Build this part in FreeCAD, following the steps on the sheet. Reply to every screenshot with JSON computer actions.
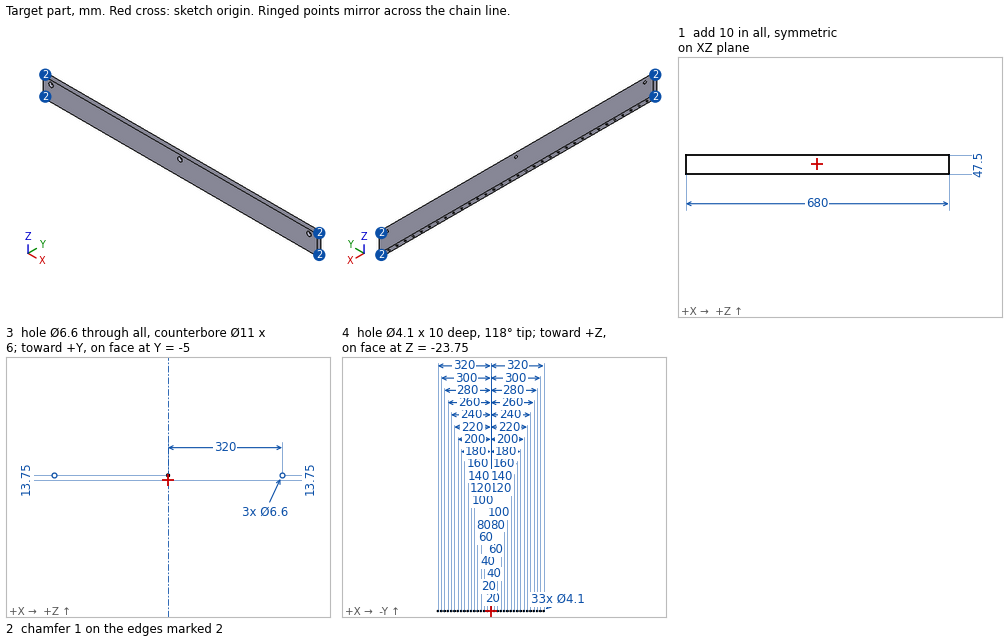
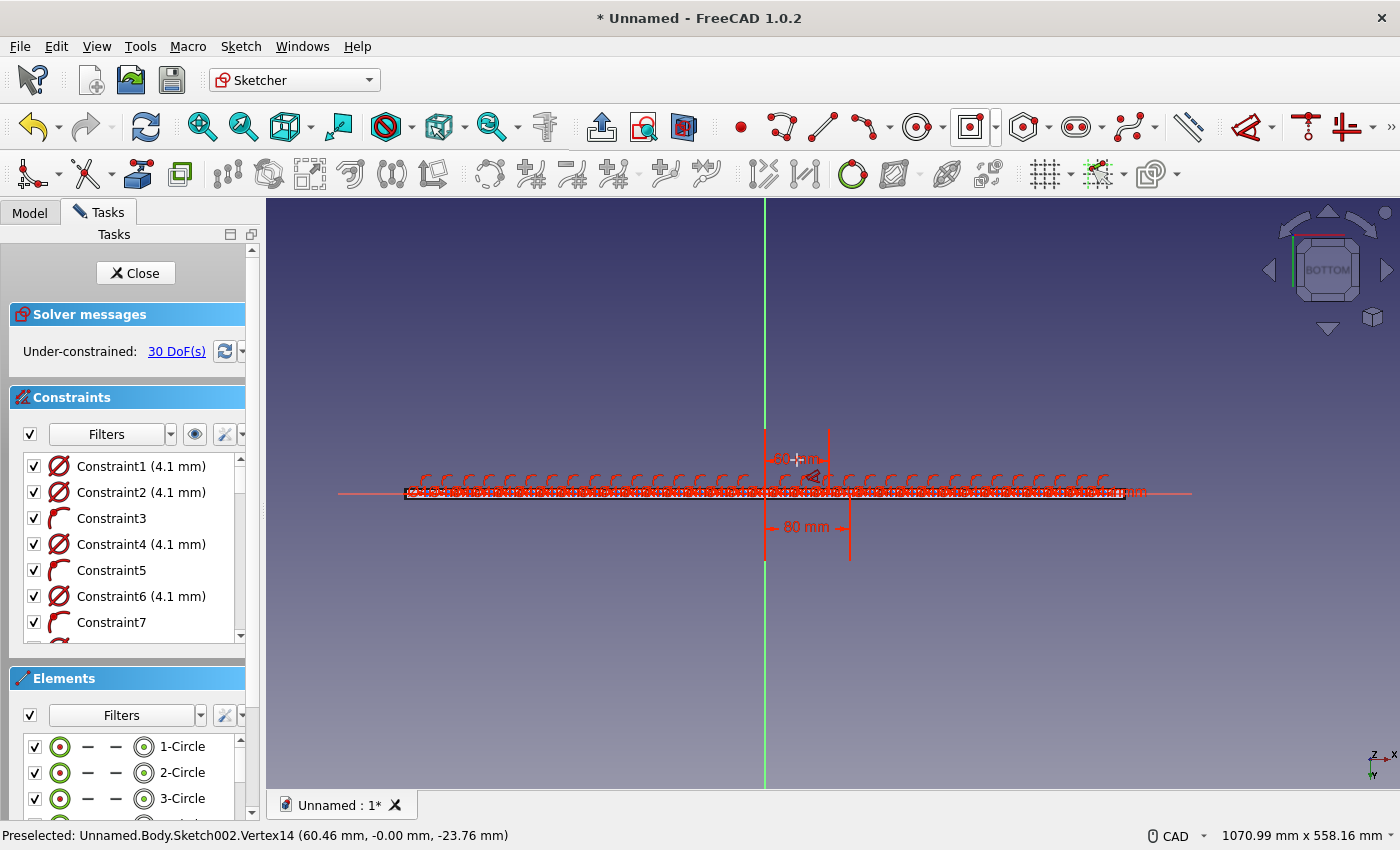
{"action": "left_click", "coordinate": [807, 494]}
{"action": "left_click", "coordinate": [786, 552]}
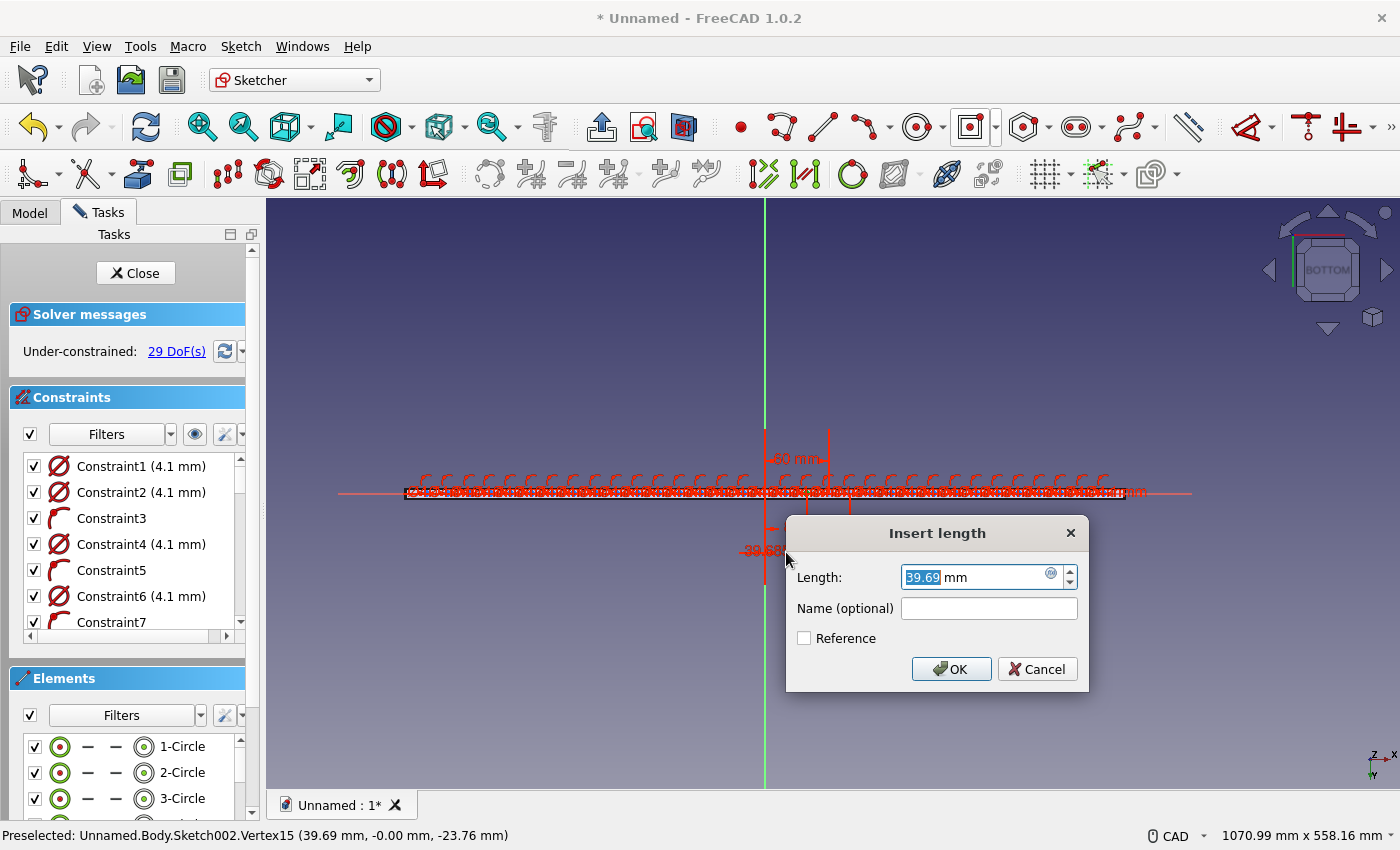
{"action": "type", "text": "40"}
{"action": "key", "text": "Return"}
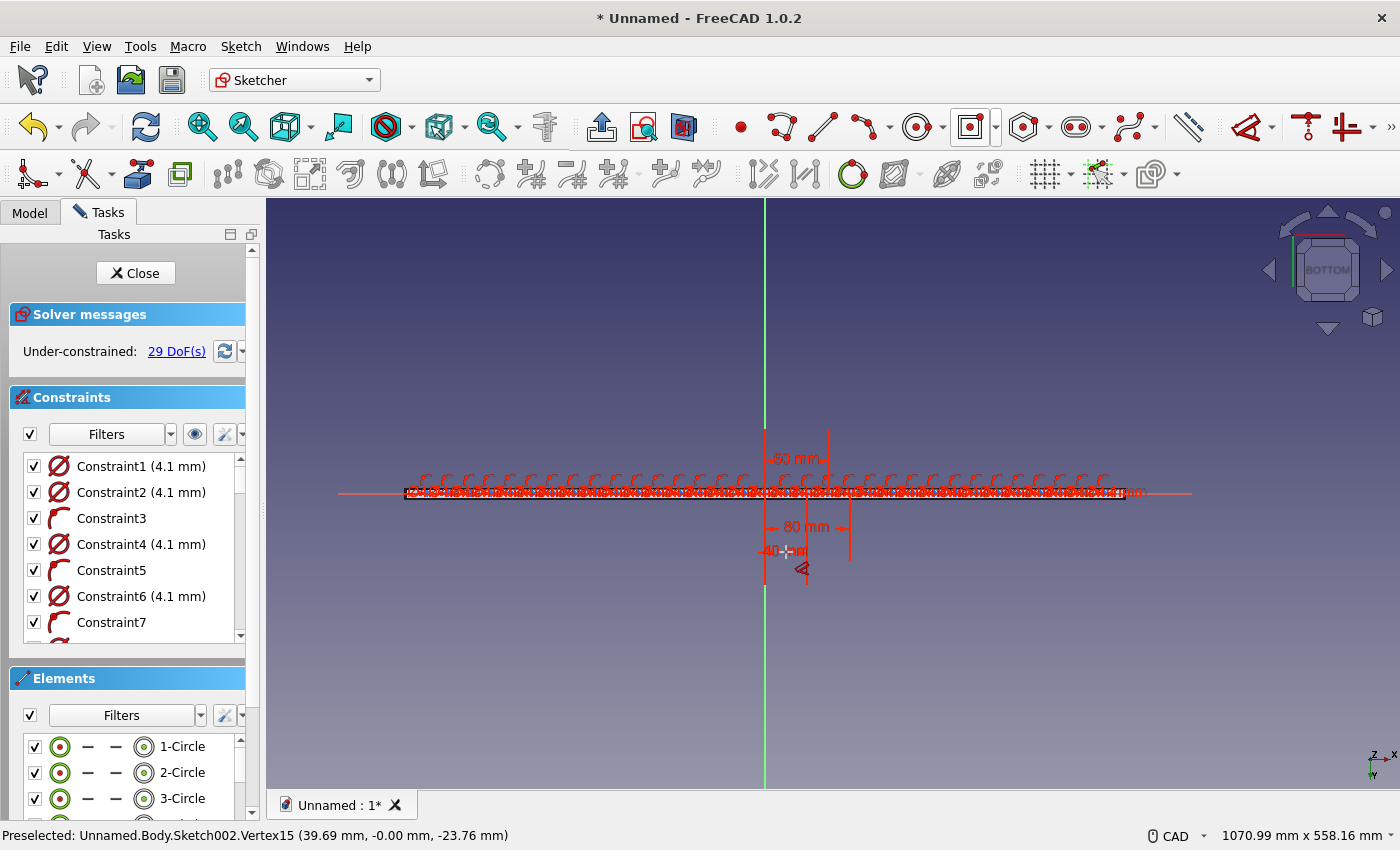
{"action": "scroll", "coordinate": [786, 494], "scroll_direction": "up", "scroll_amount": 4}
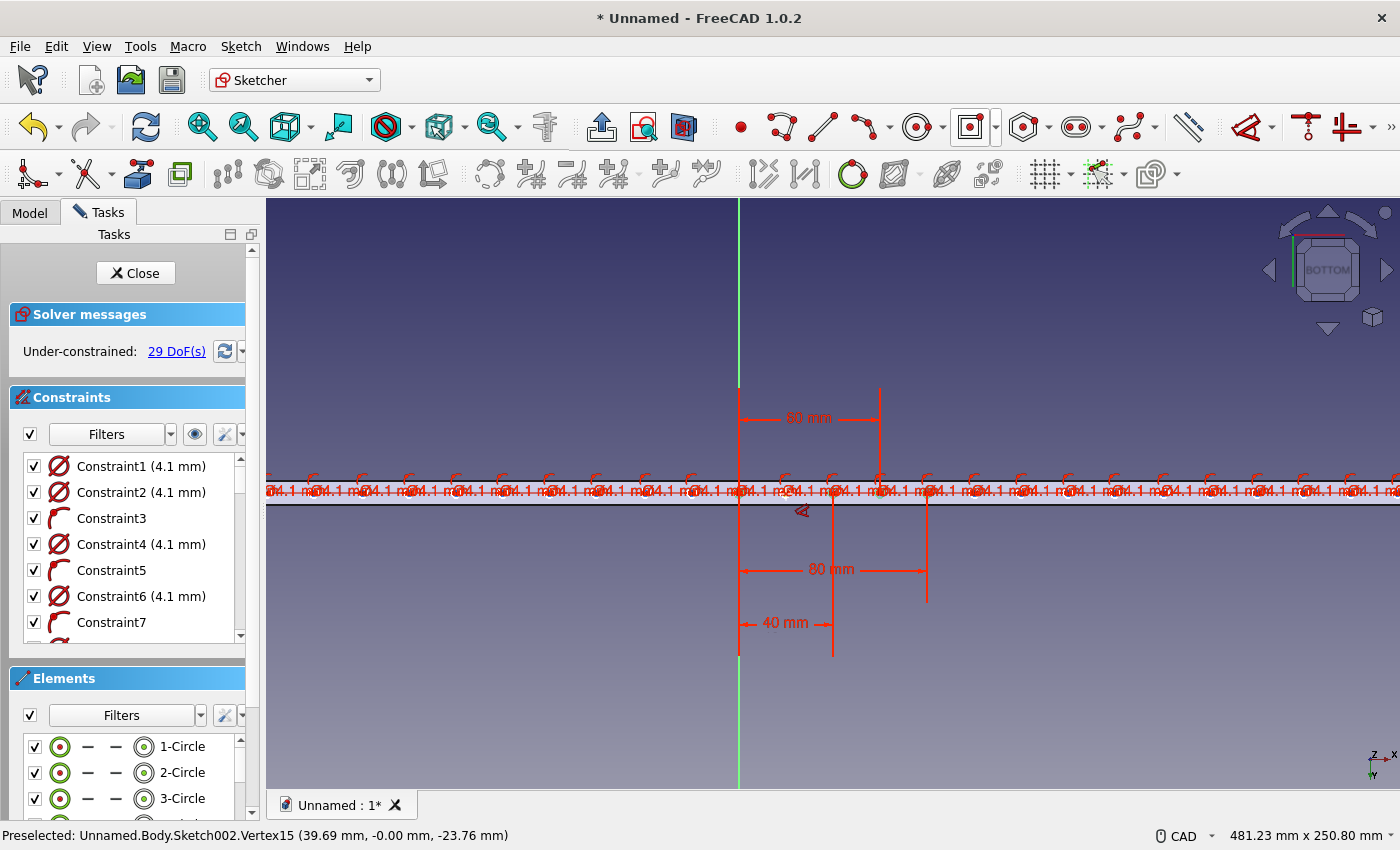
{"action": "left_click", "coordinate": [785, 493]}
{"action": "left_click", "coordinate": [762, 527]}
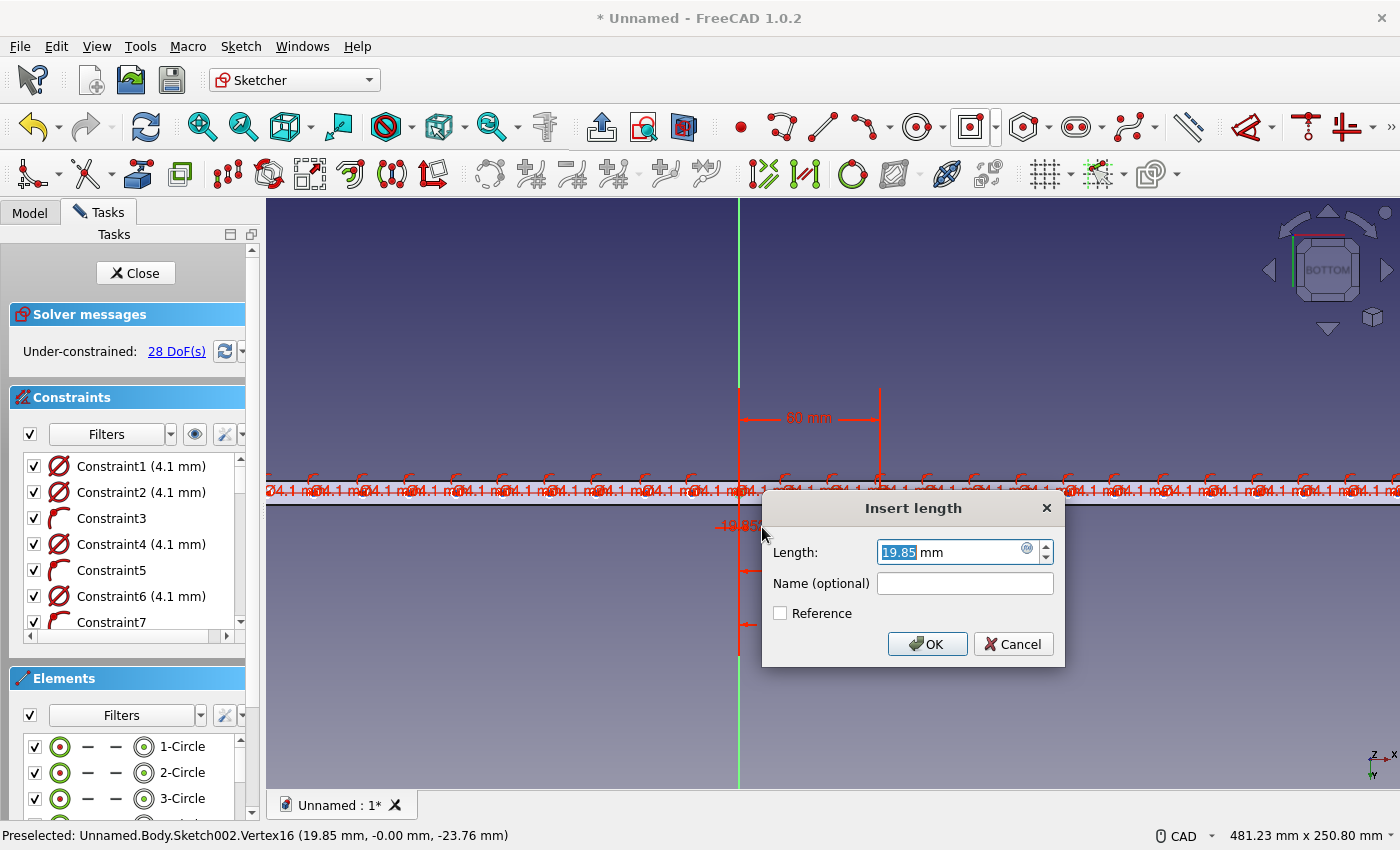
{"action": "type", "text": "20"}
{"action": "key", "text": "Return"}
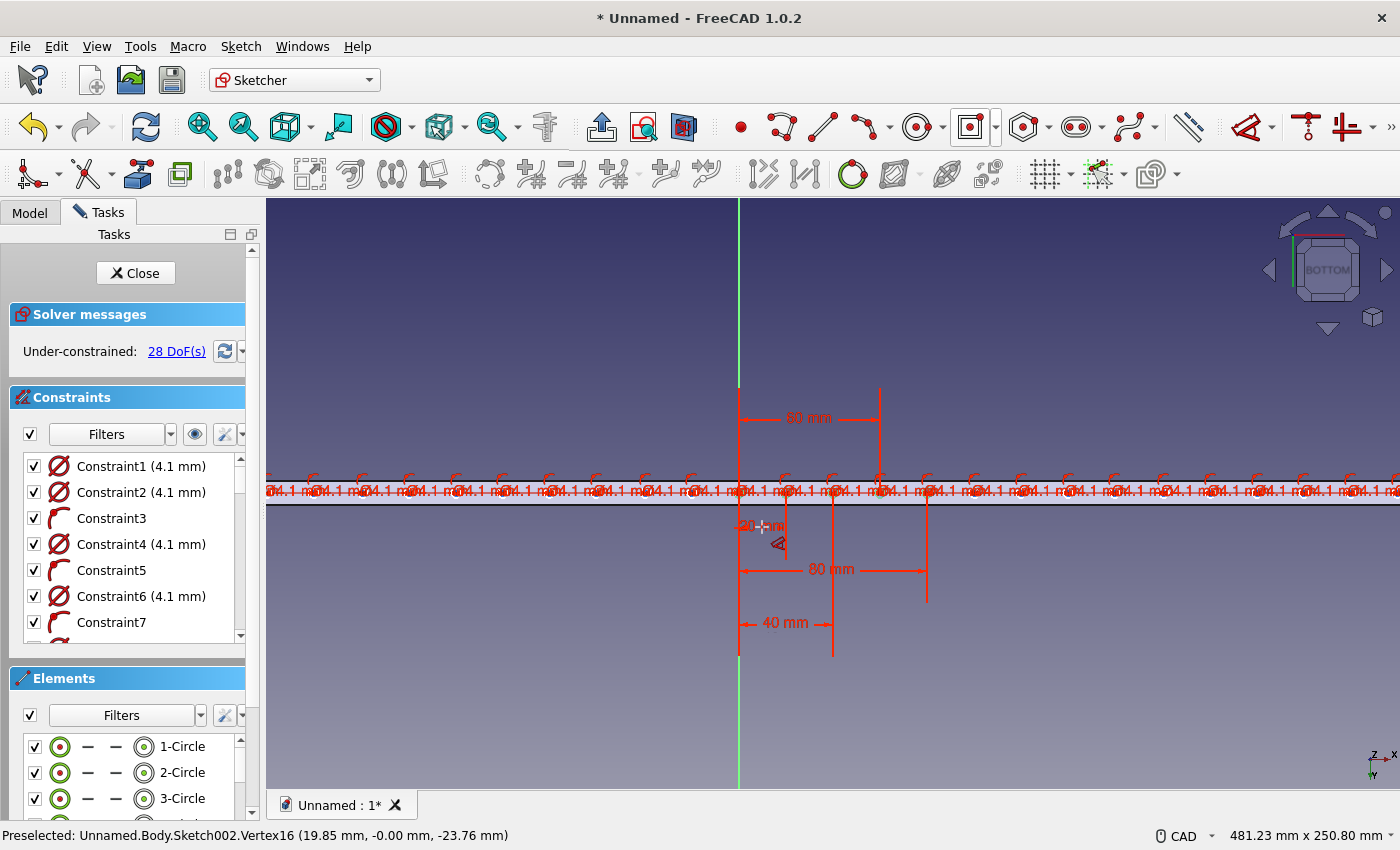
{"action": "left_click", "coordinate": [692, 493]}
{"action": "left_click", "coordinate": [715, 459]}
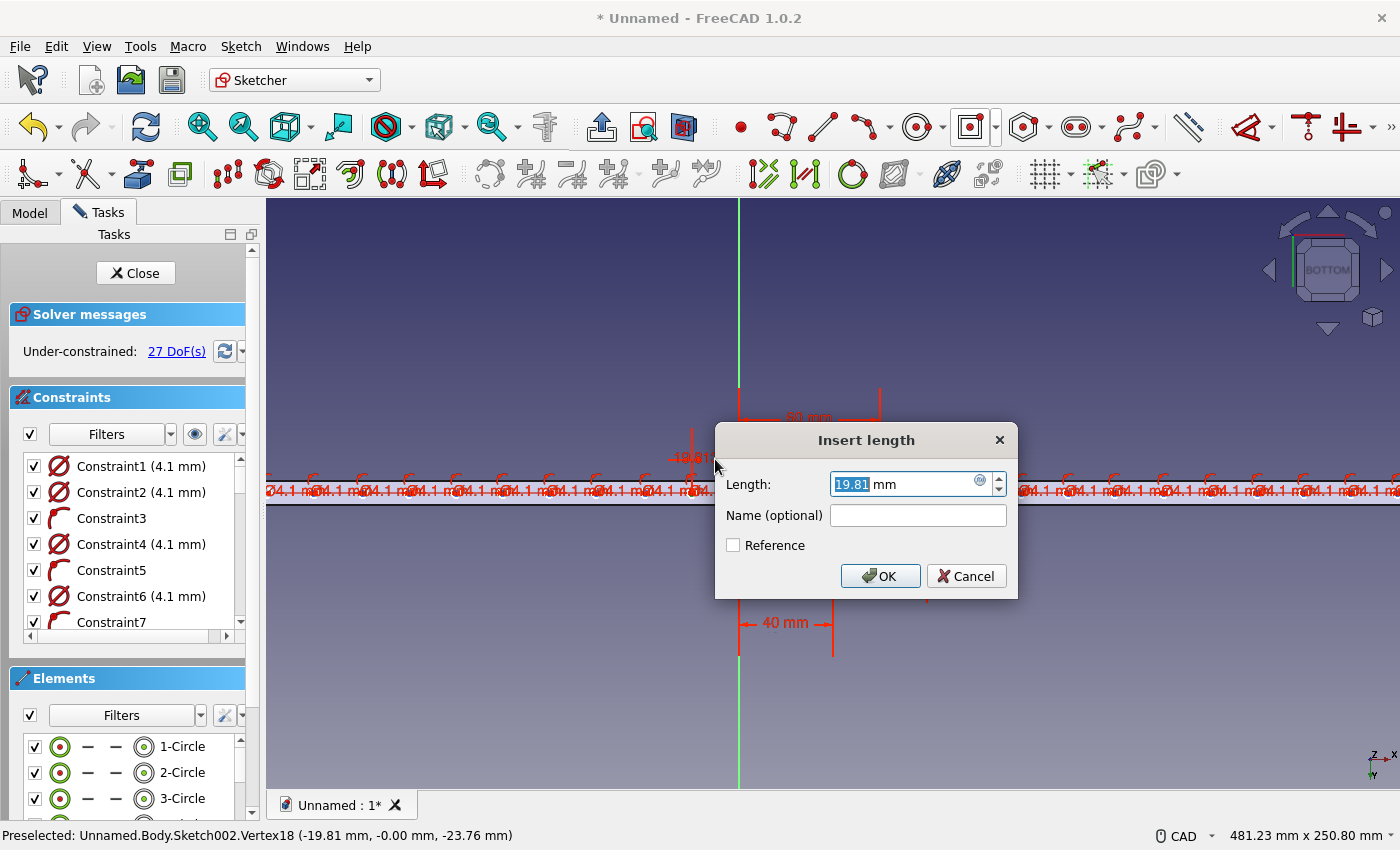
{"action": "type", "text": "20"}
{"action": "key", "text": "Return"}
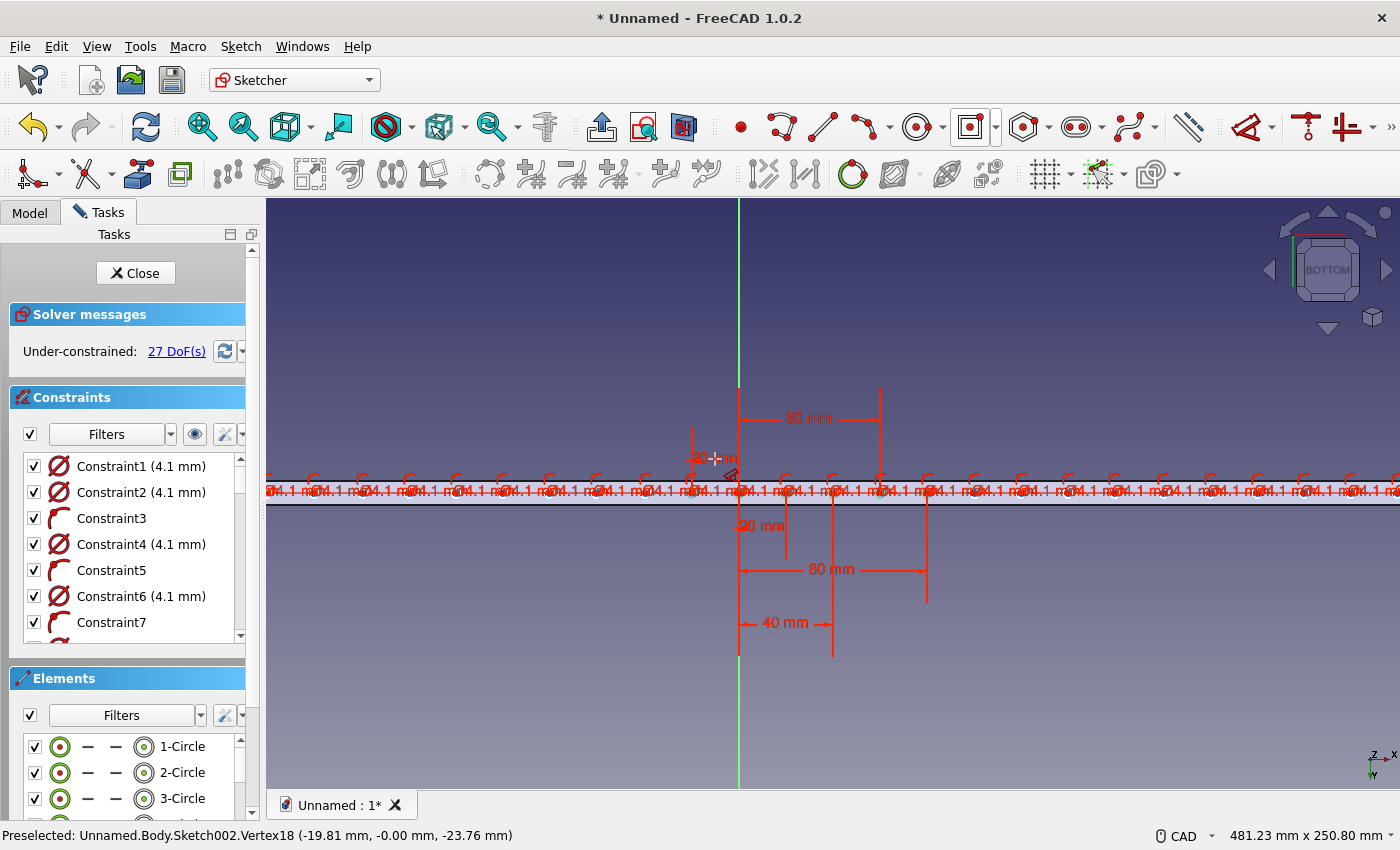
{"action": "left_click", "coordinate": [645, 493]}
{"action": "left_click", "coordinate": [692, 527]}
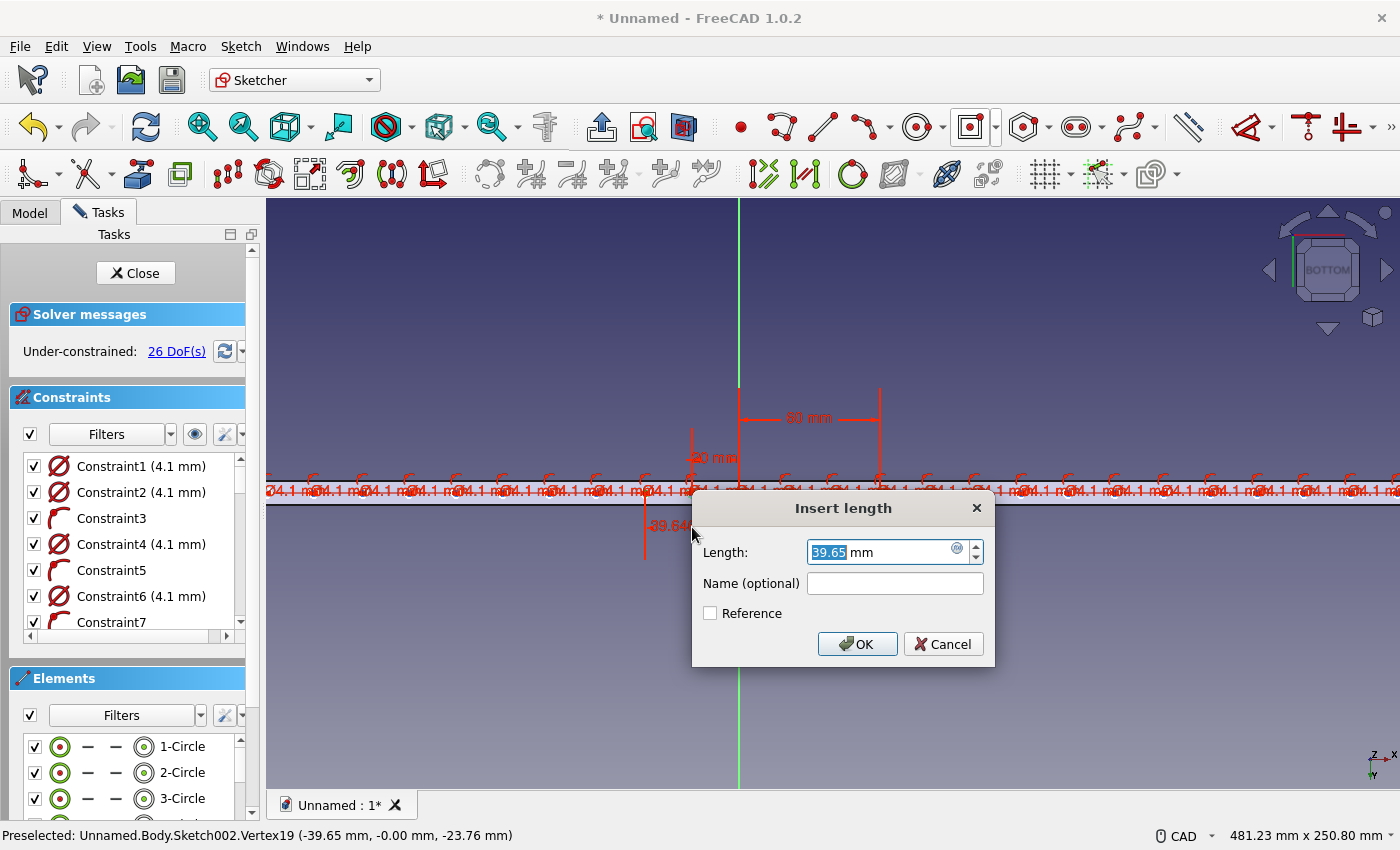
{"action": "type", "text": "40"}
{"action": "key", "text": "Return"}